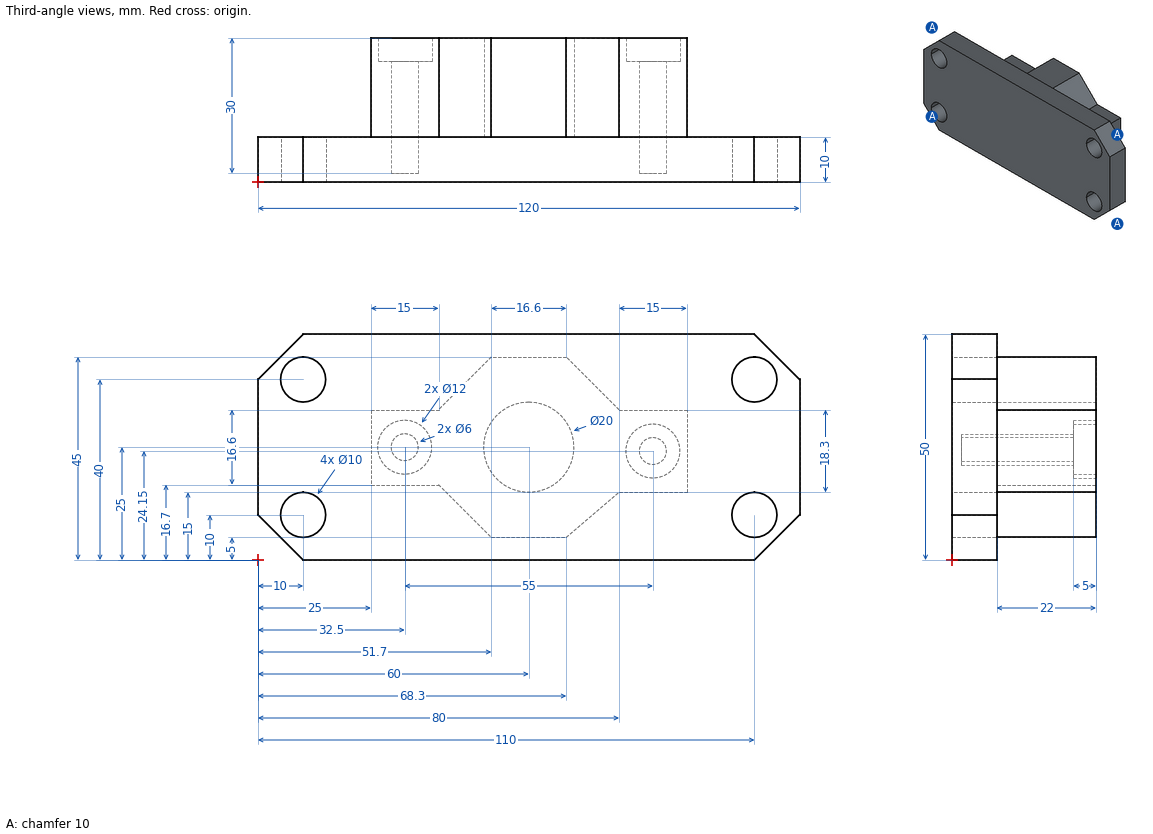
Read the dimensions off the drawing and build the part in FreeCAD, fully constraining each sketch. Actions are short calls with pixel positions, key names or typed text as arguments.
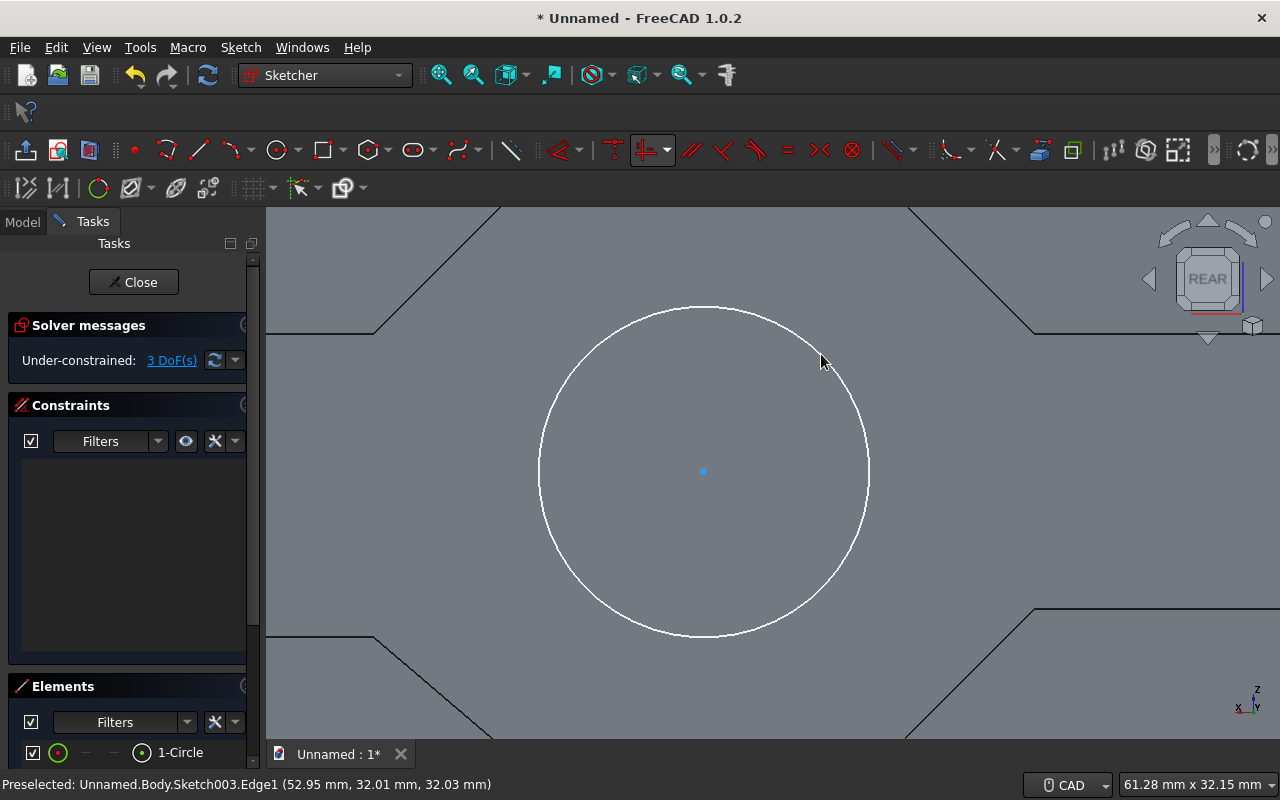
click(558, 150)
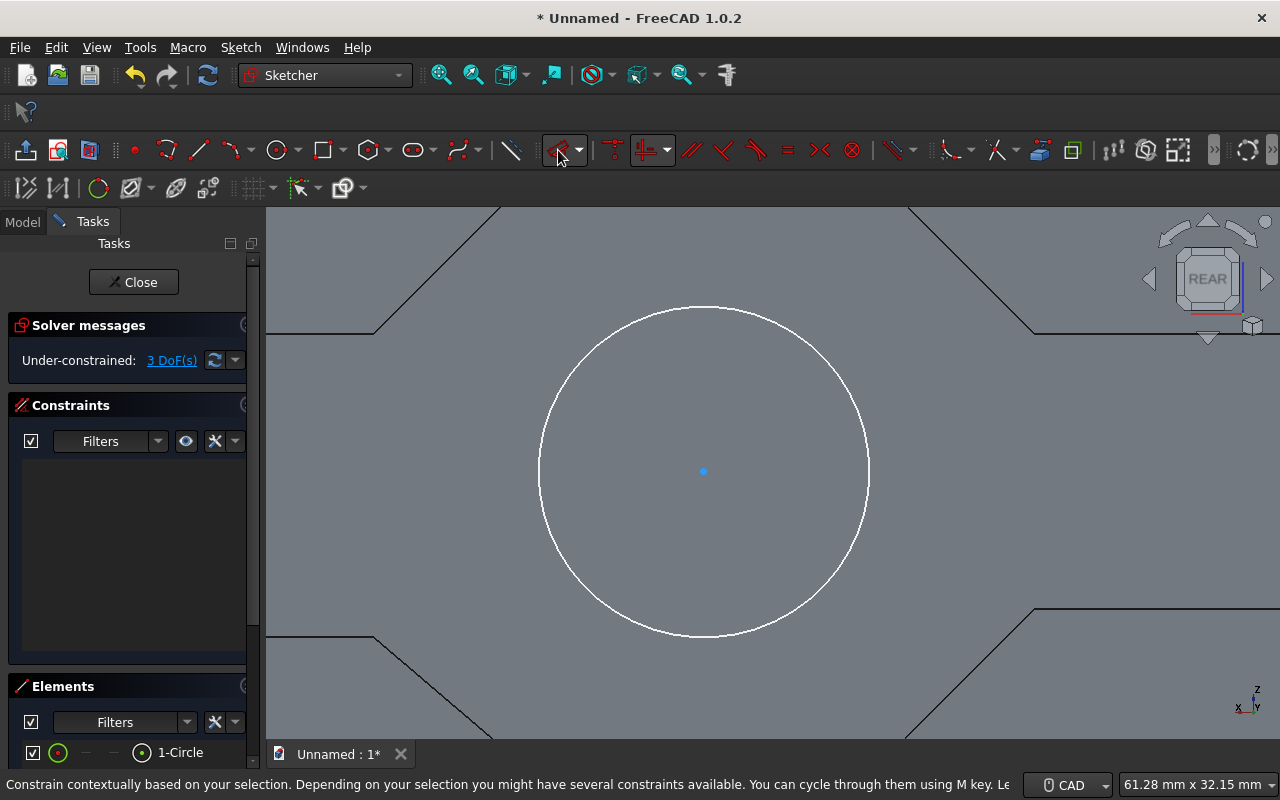
click(821, 355)
click(844, 332)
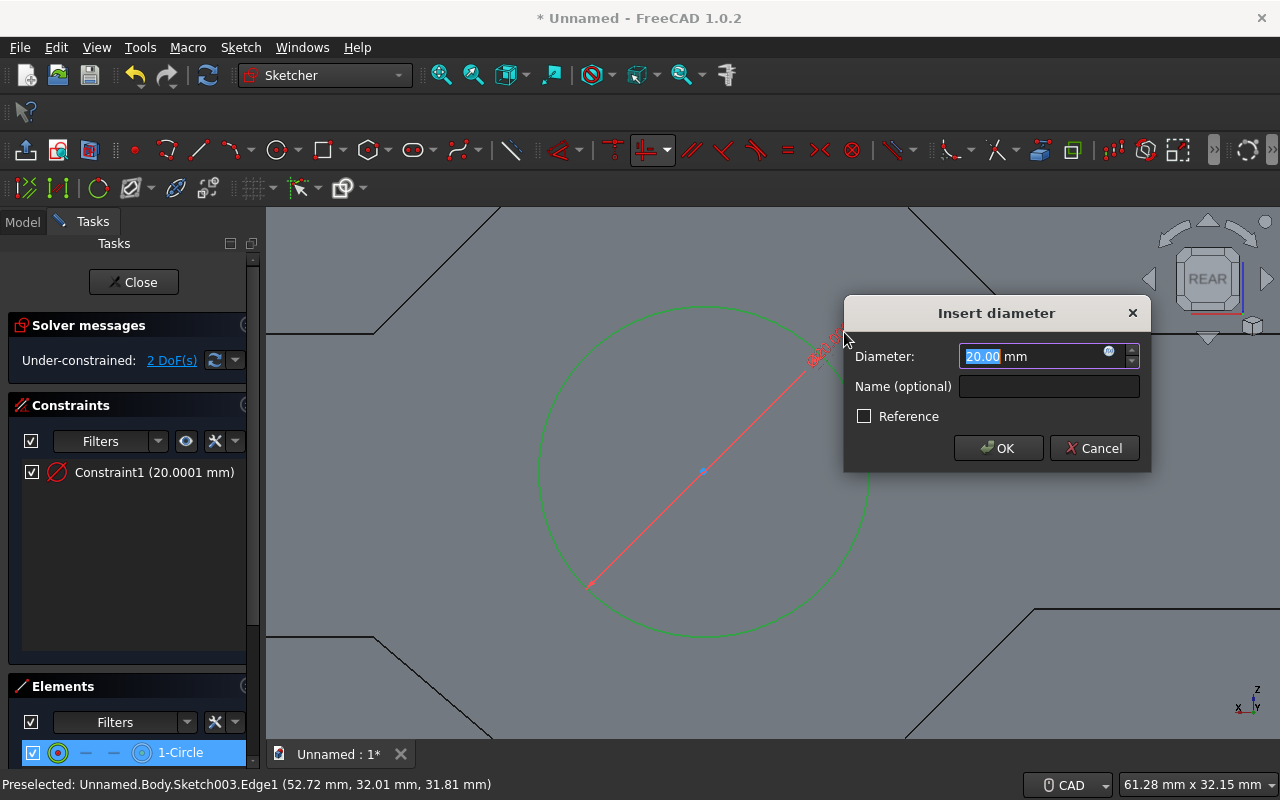
text(20)
key(Return)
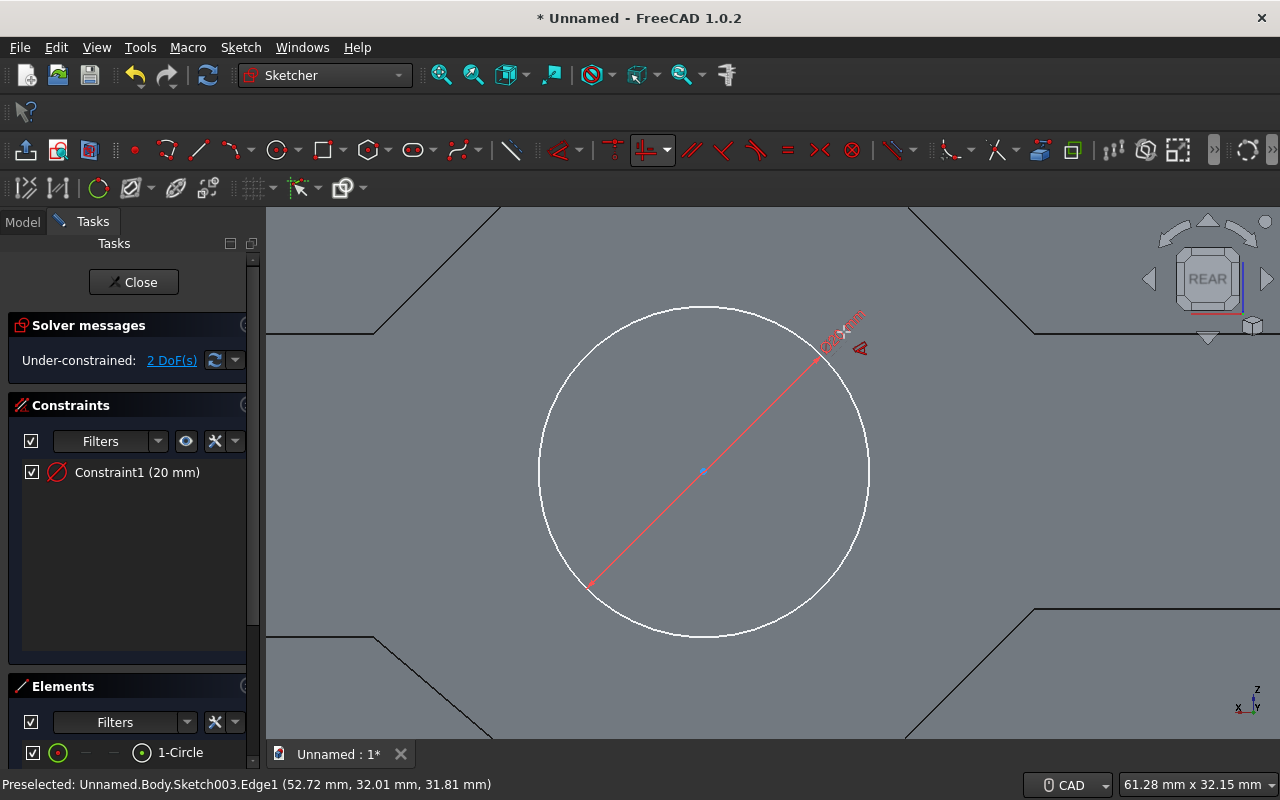
click(704, 472)
click(910, 438)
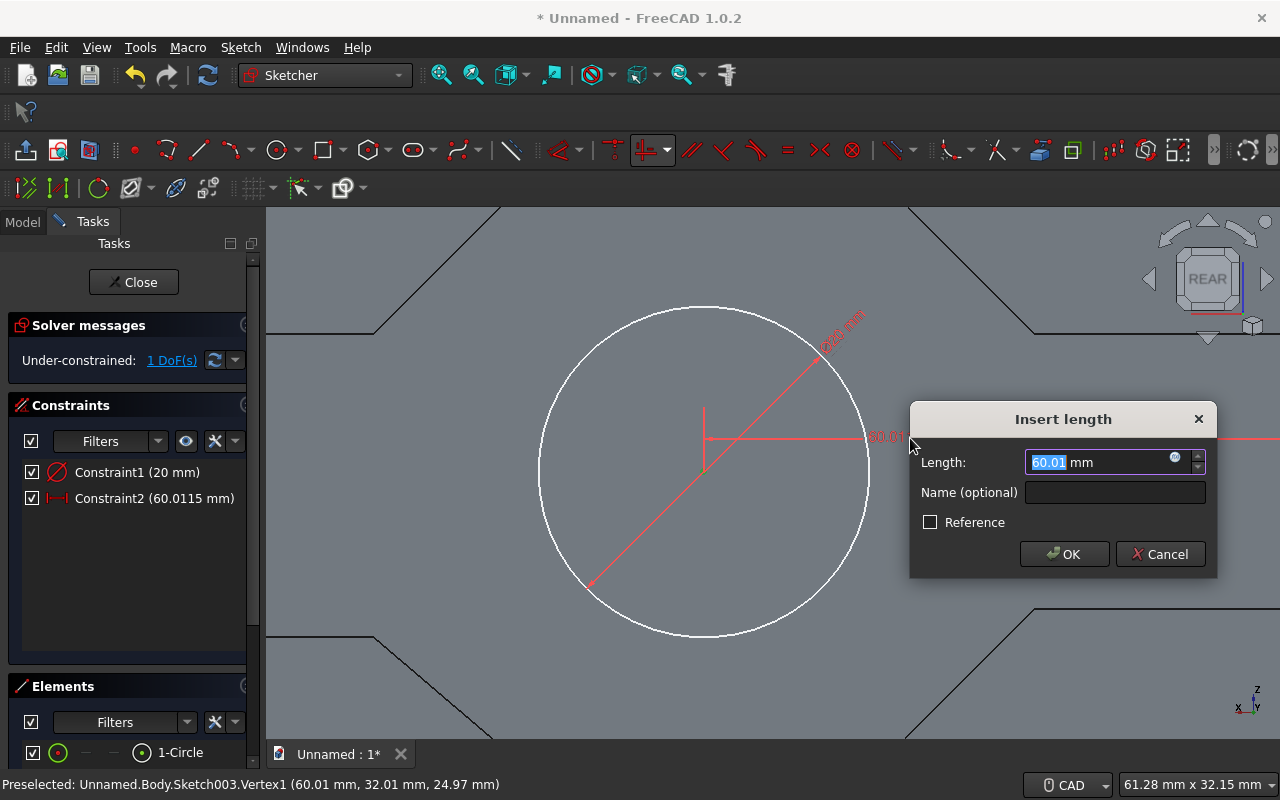
text(60)
key(Return)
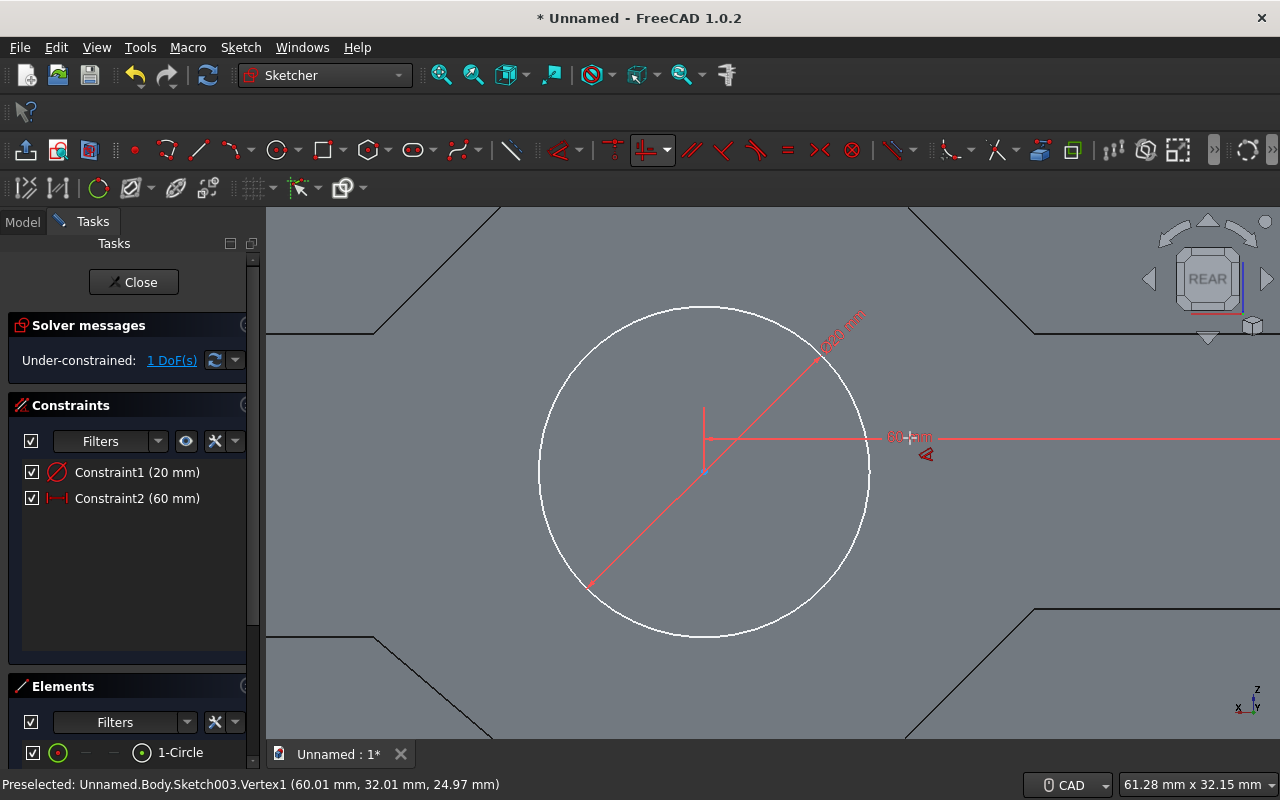
click(704, 472)
click(670, 592)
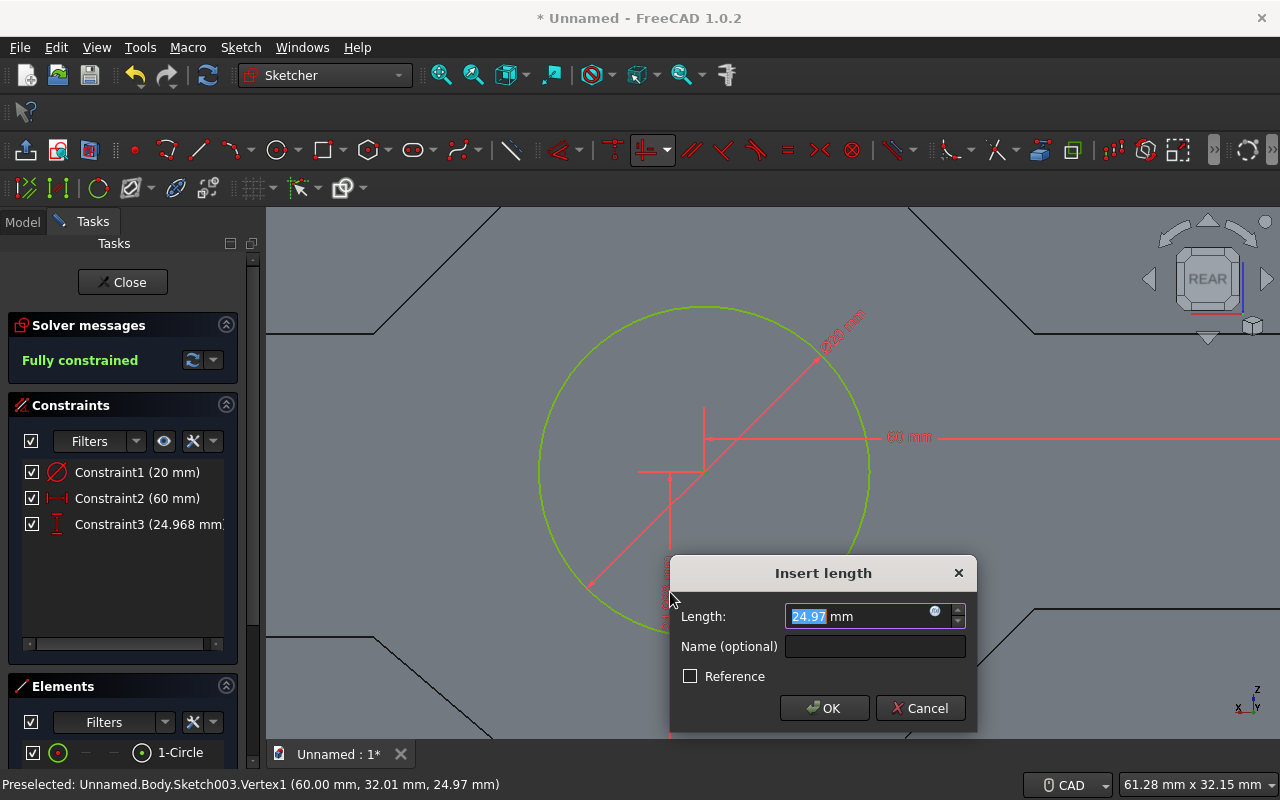
text(25)
key(Return)
key(Escape)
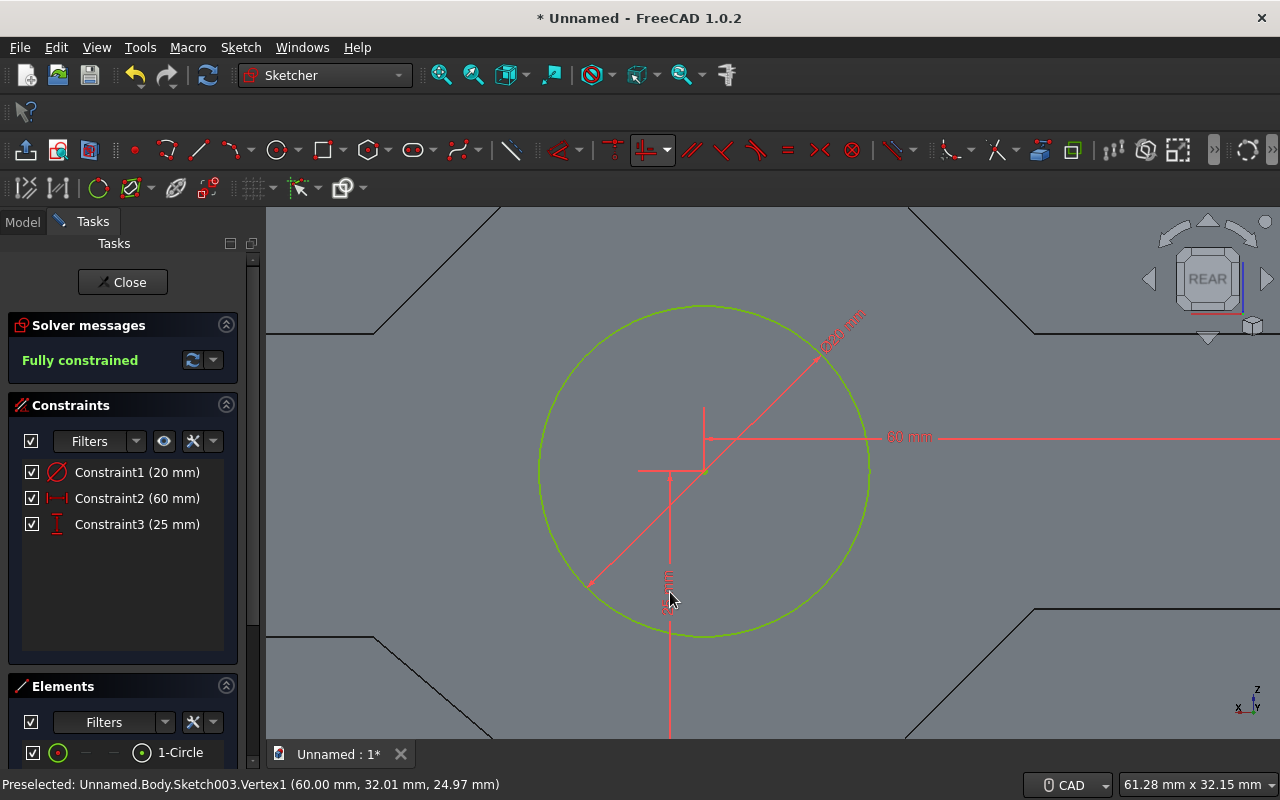
click(123, 282)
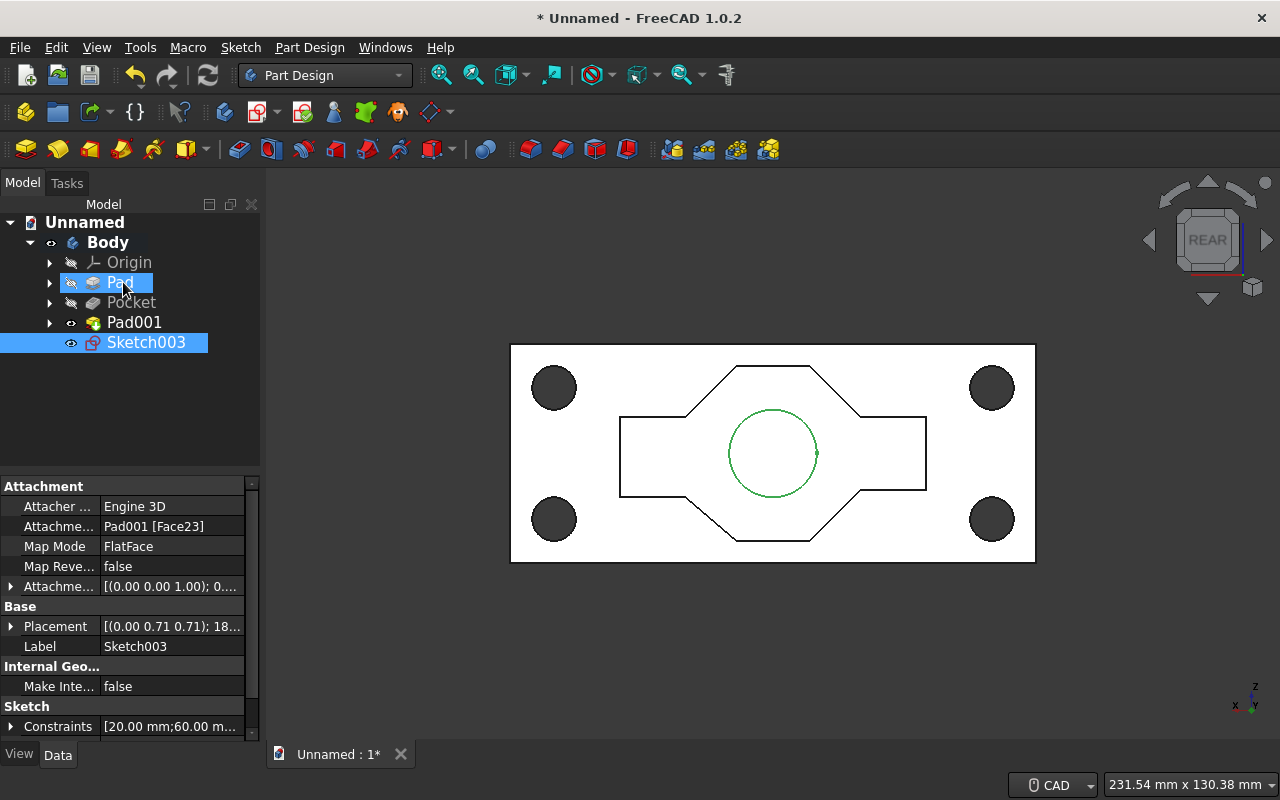
click(240, 150)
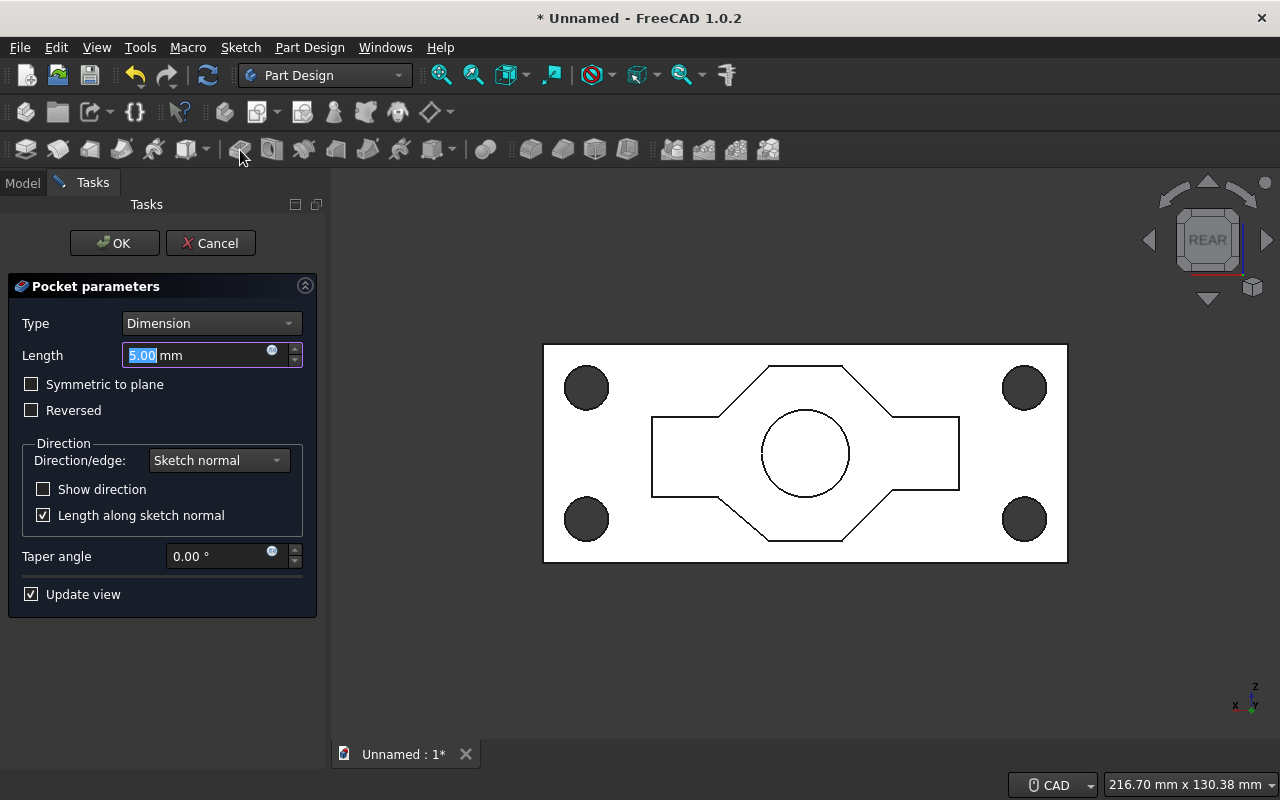
text(22)
key(Tab)